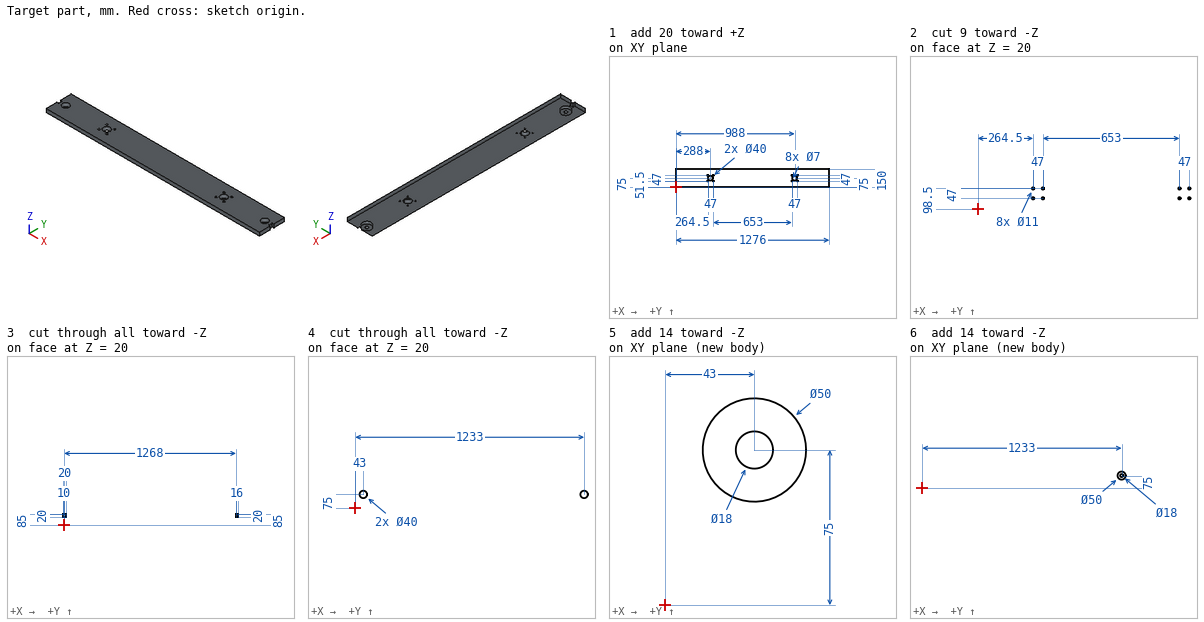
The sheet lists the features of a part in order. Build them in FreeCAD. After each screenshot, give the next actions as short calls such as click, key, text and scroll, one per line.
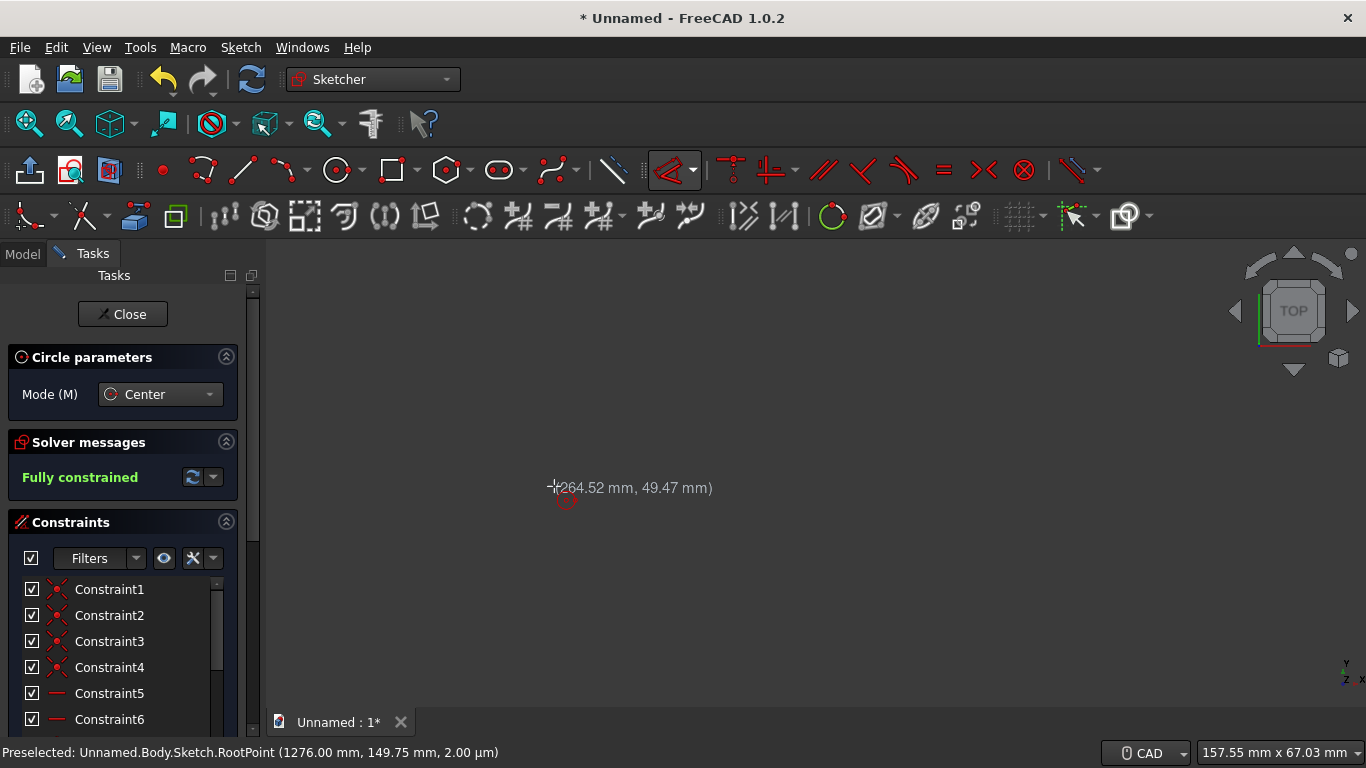
scroll(554, 486, down, 13)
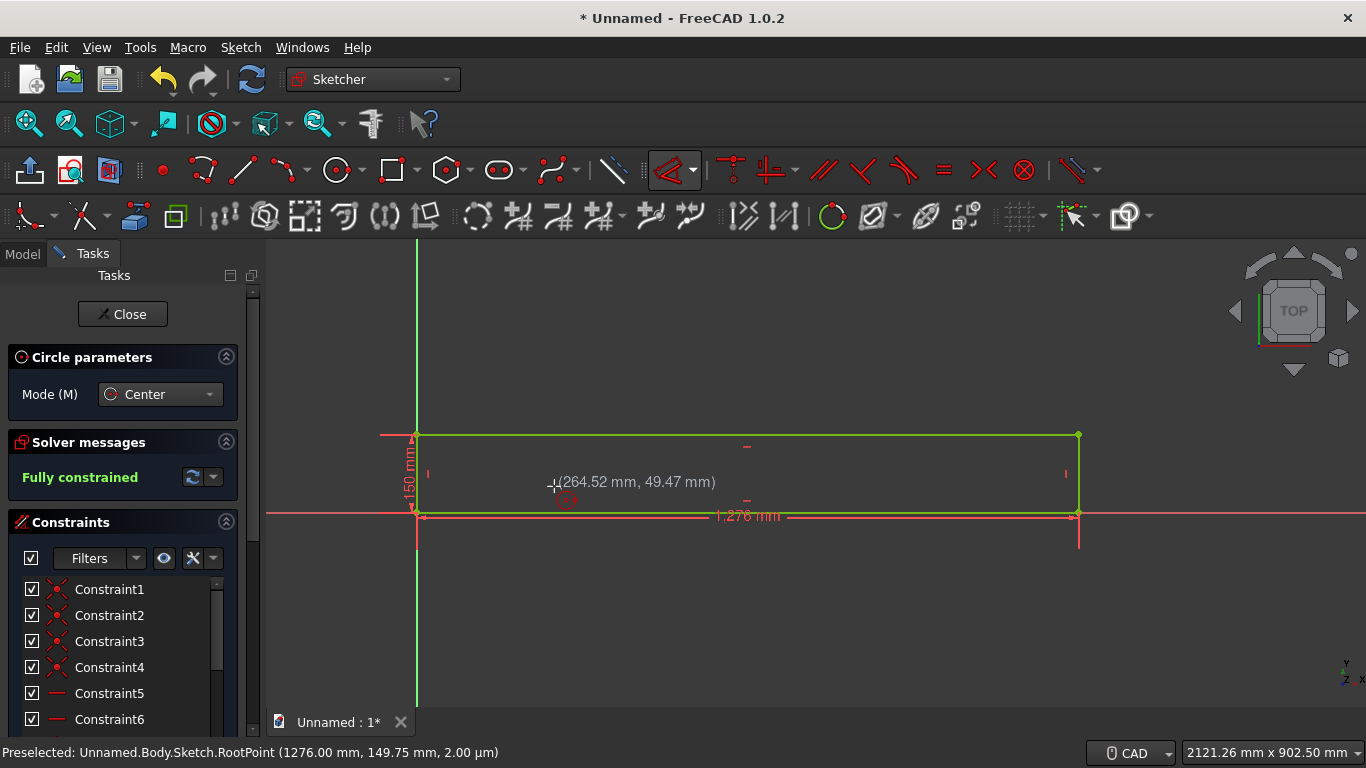
click(554, 486)
move(555, 485)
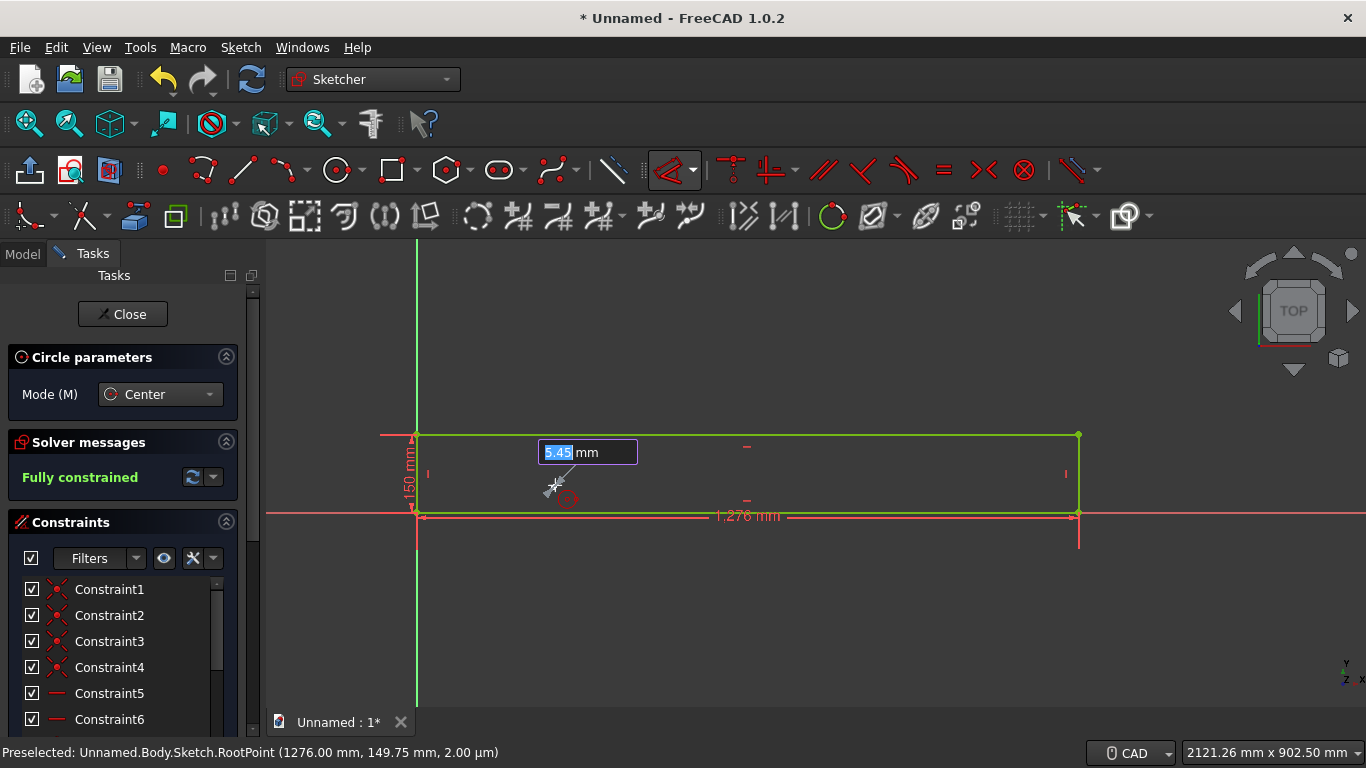
text(7)
key(Return)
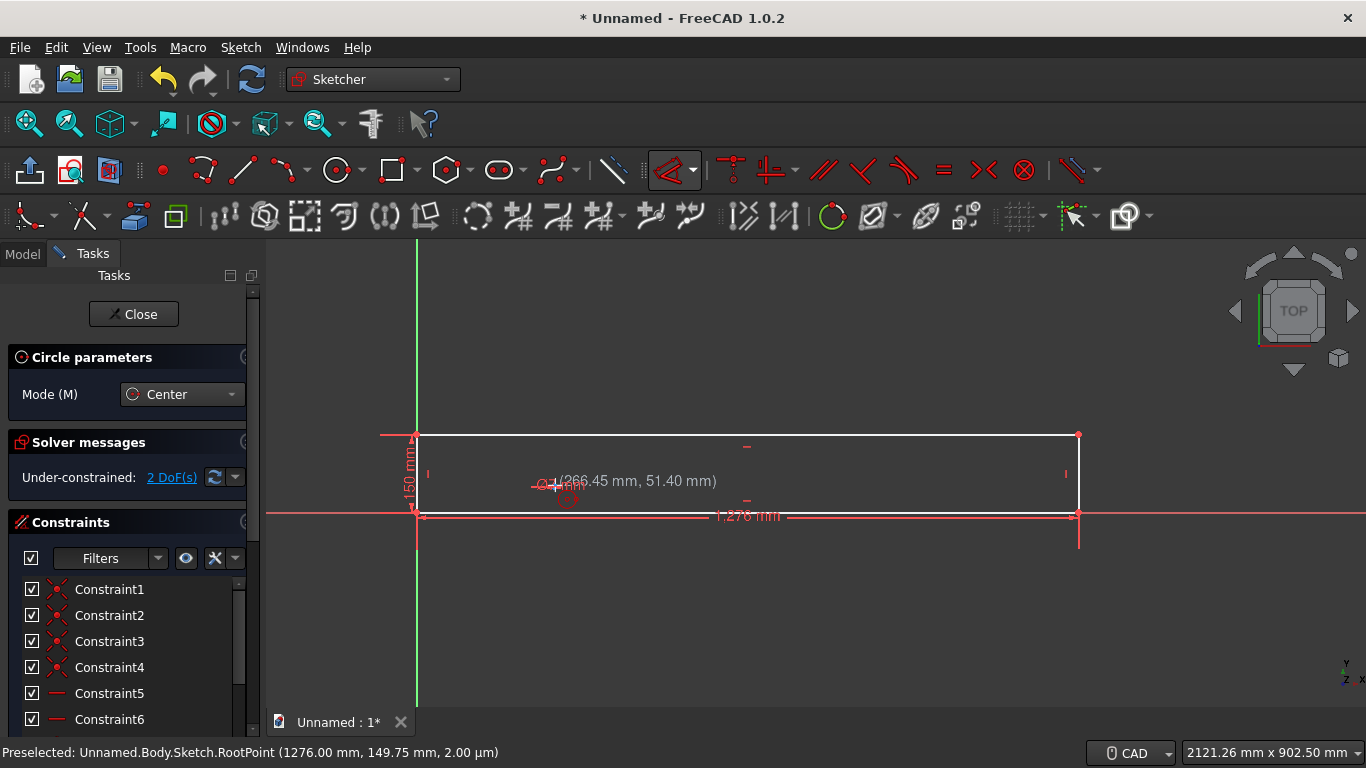
scroll(578, 486, up, 13)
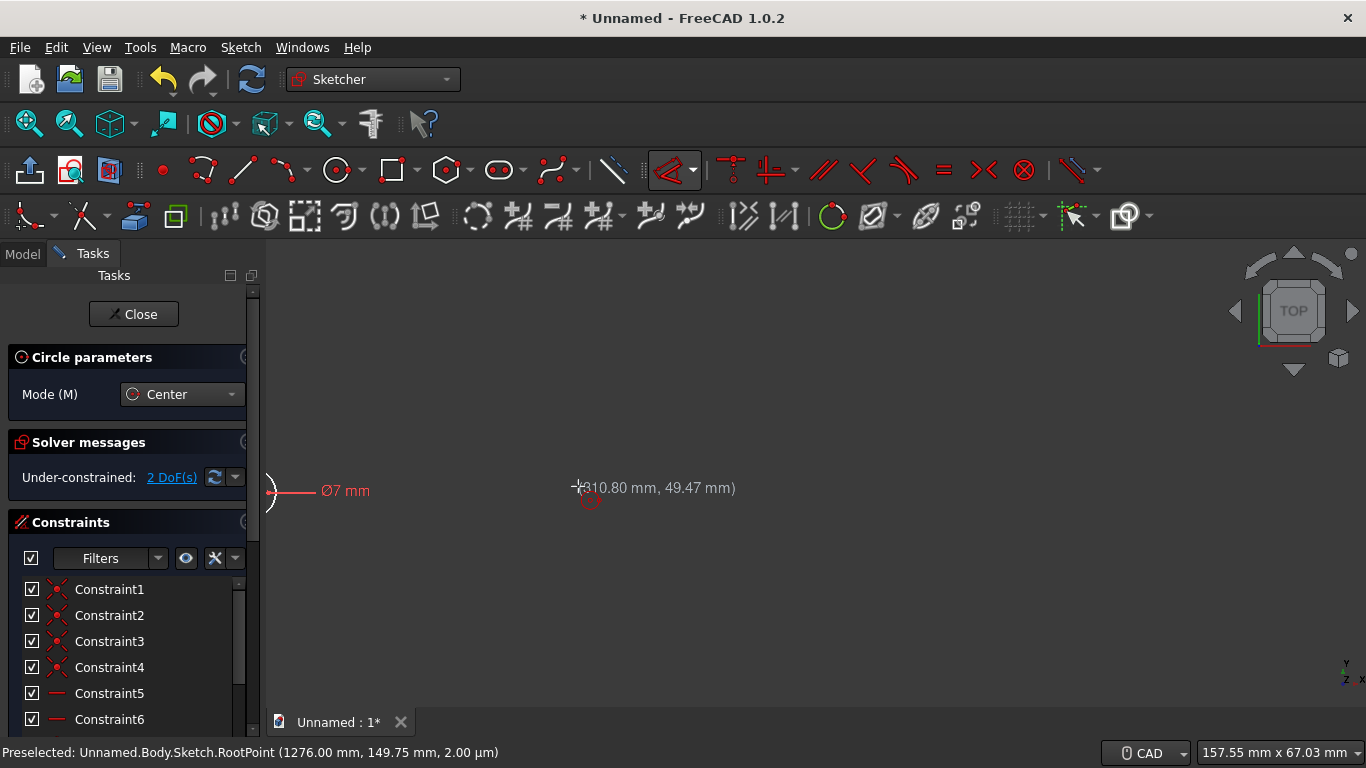
scroll(578, 486, down, 13)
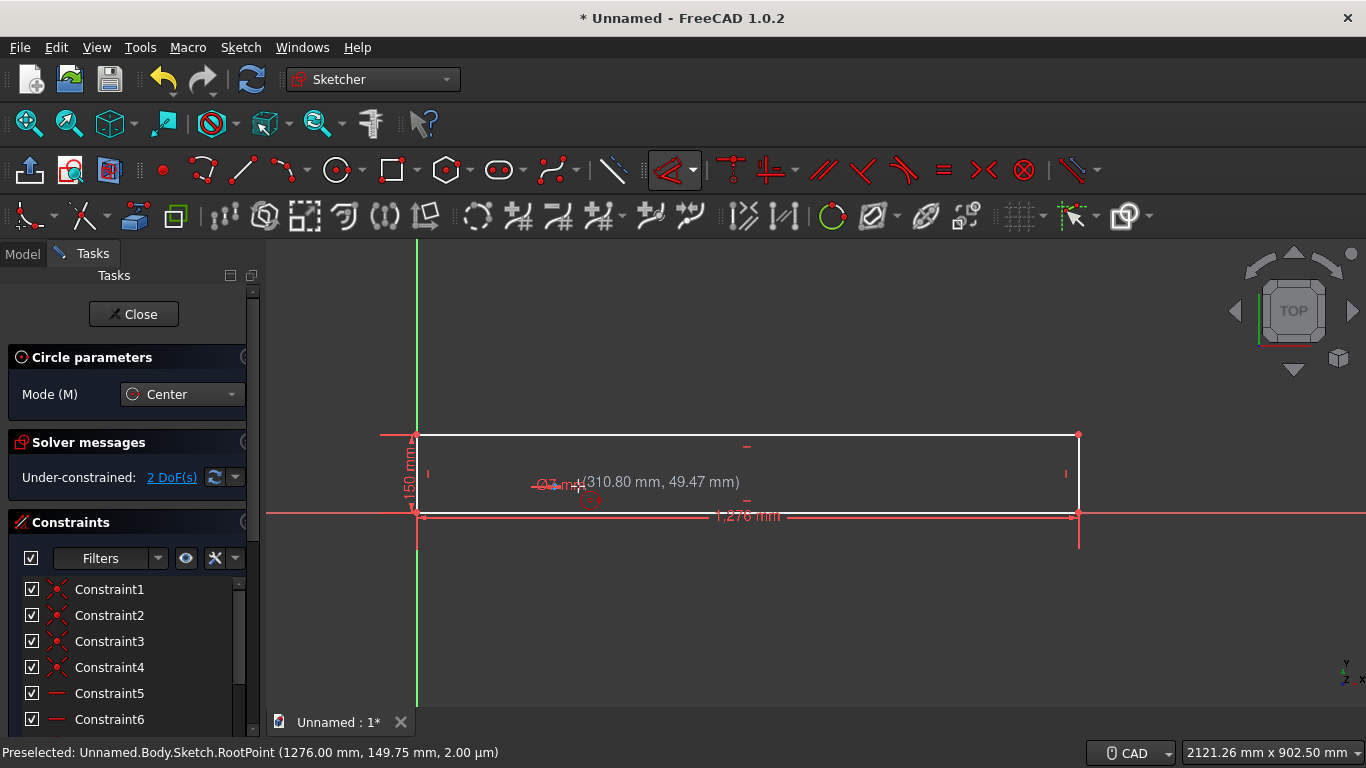
click(578, 486)
move(580, 485)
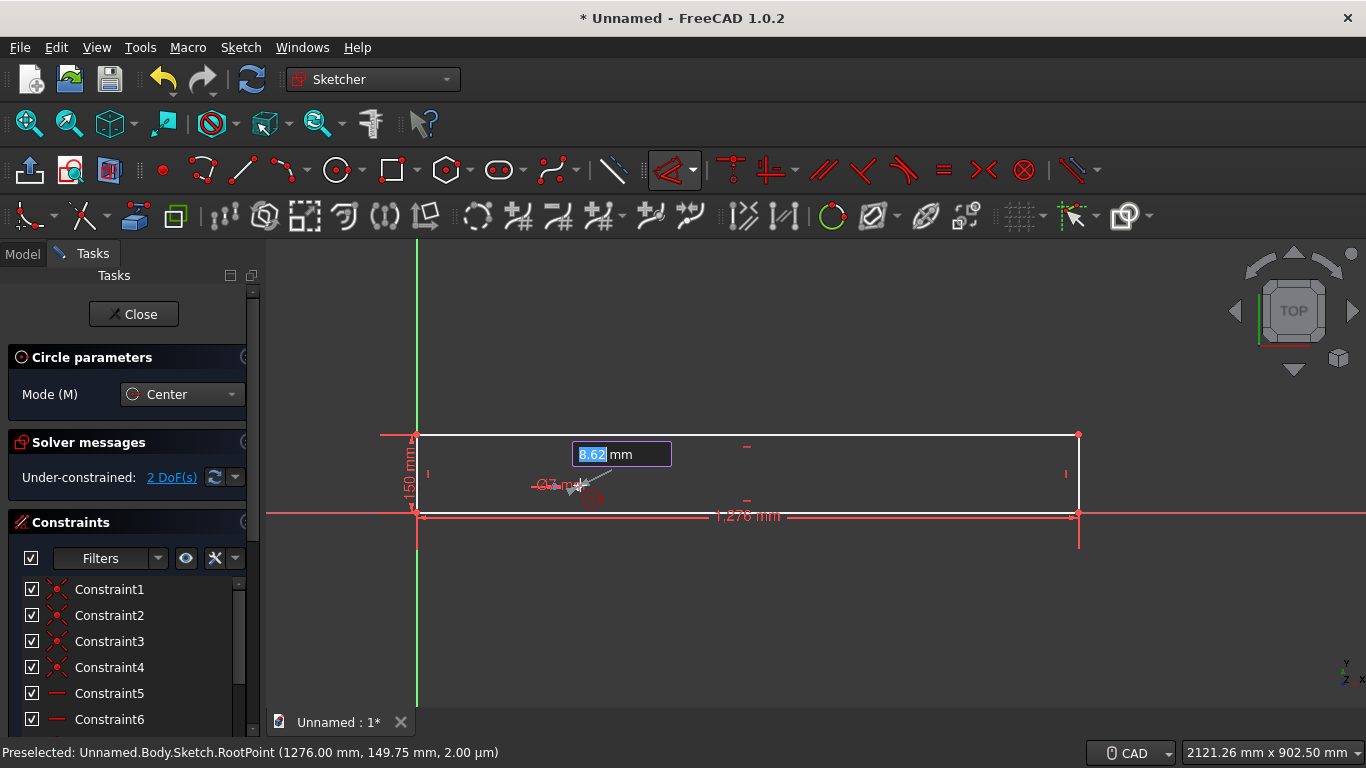
text(7)
key(Return)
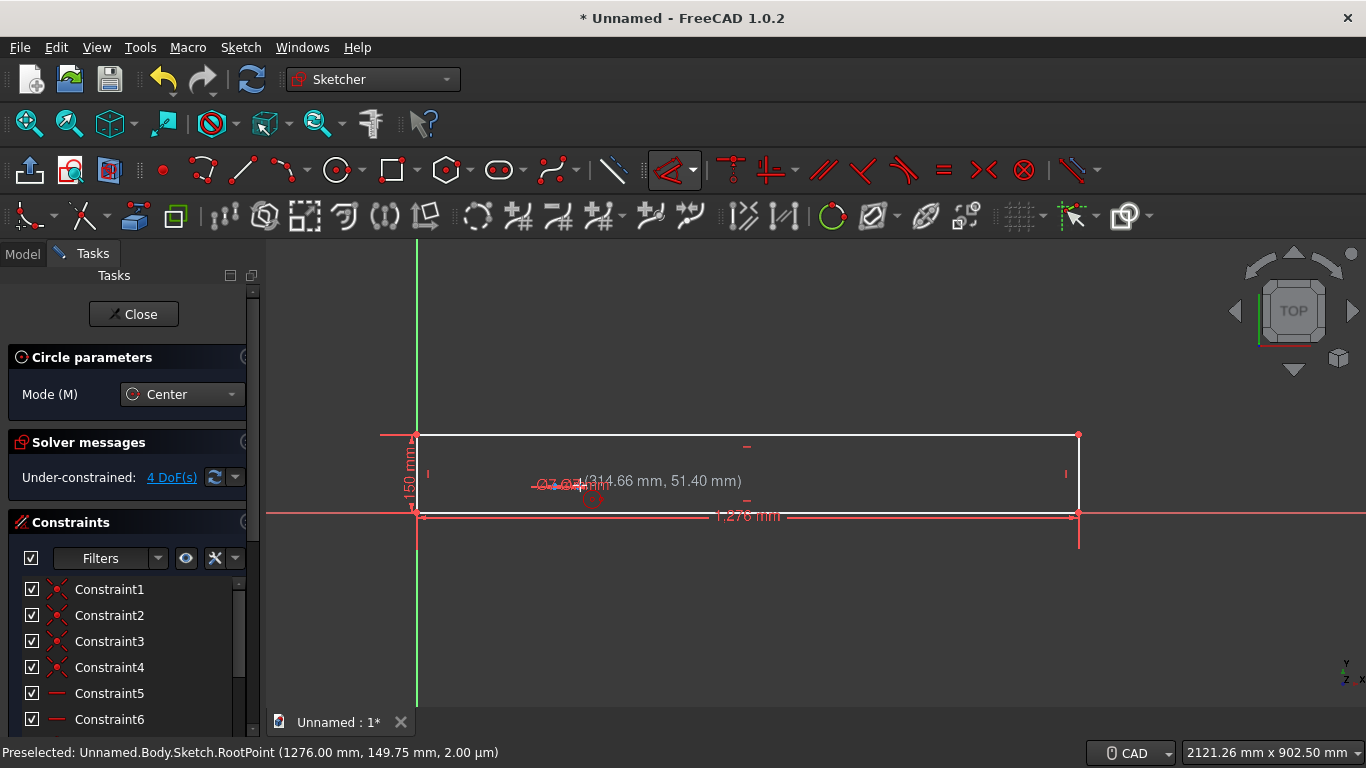
scroll(917, 486, up, 13)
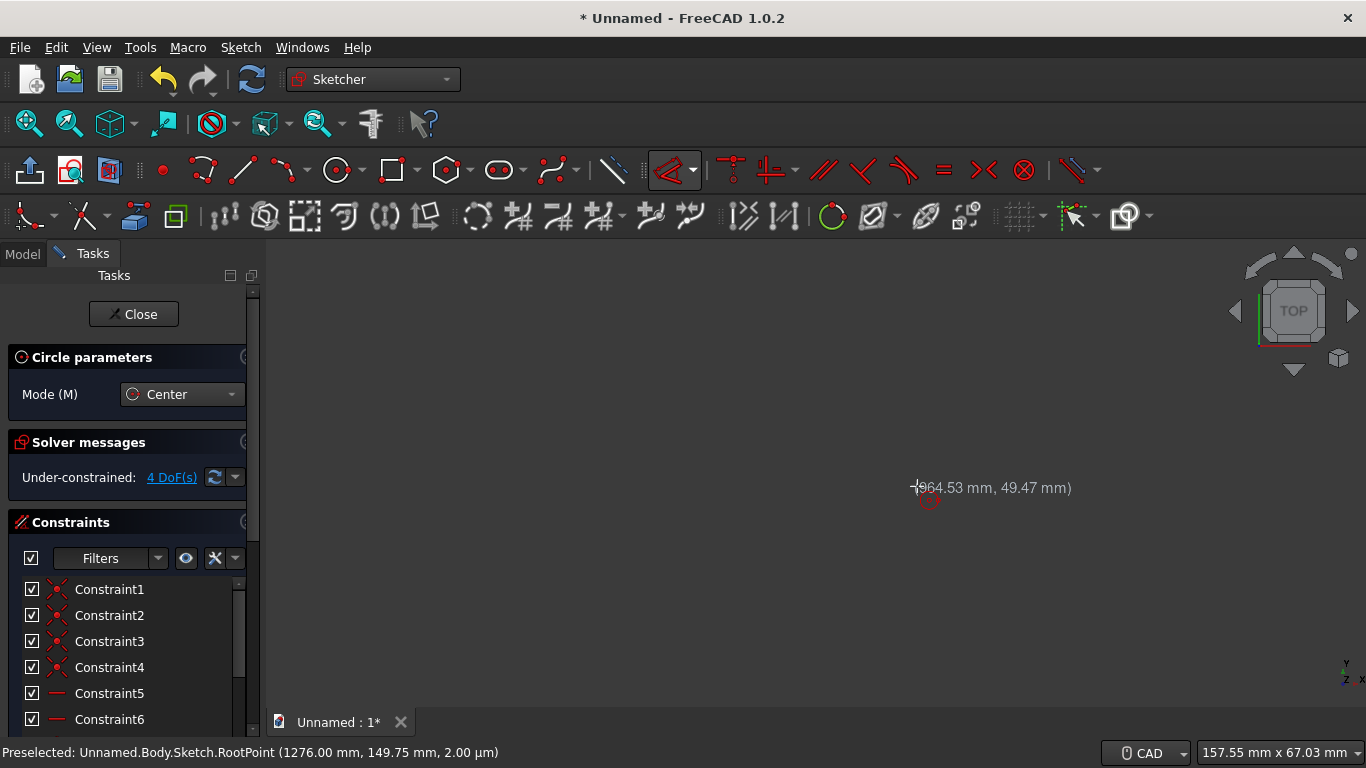
scroll(917, 486, down, 13)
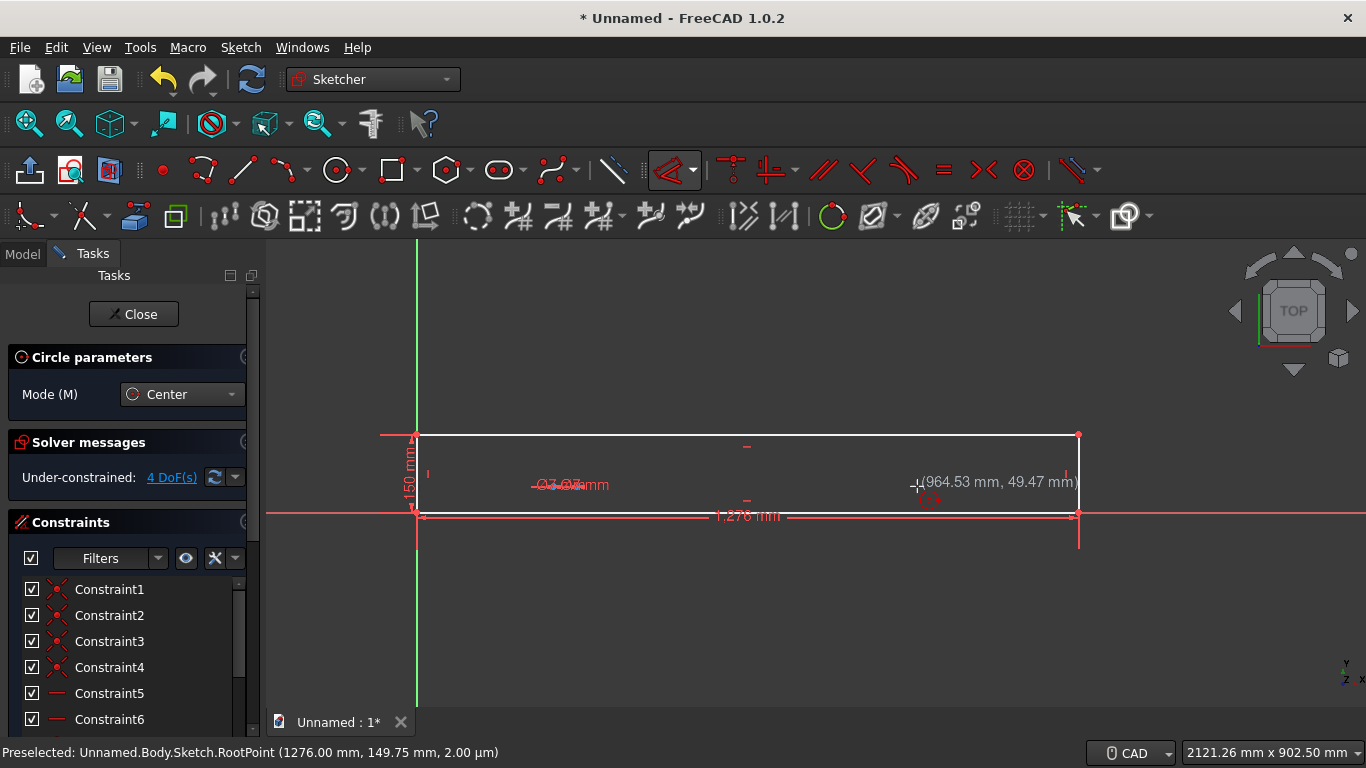
click(917, 486)
move(918, 485)